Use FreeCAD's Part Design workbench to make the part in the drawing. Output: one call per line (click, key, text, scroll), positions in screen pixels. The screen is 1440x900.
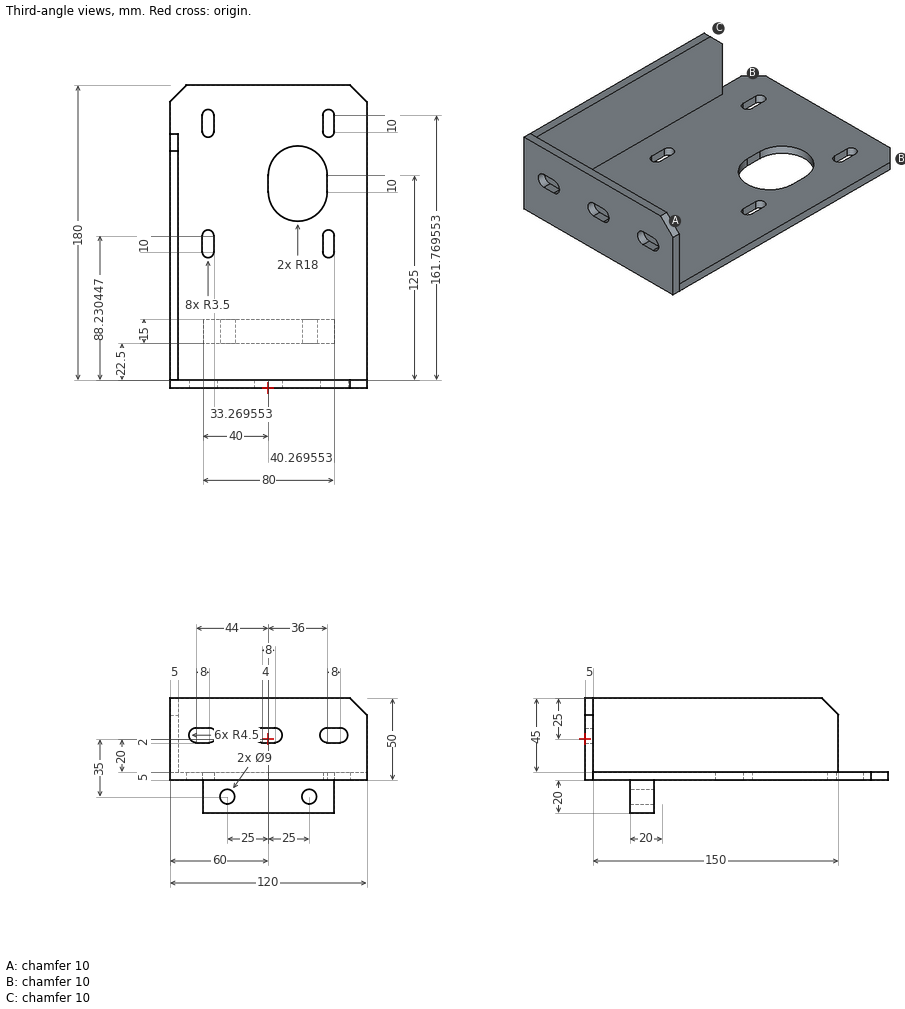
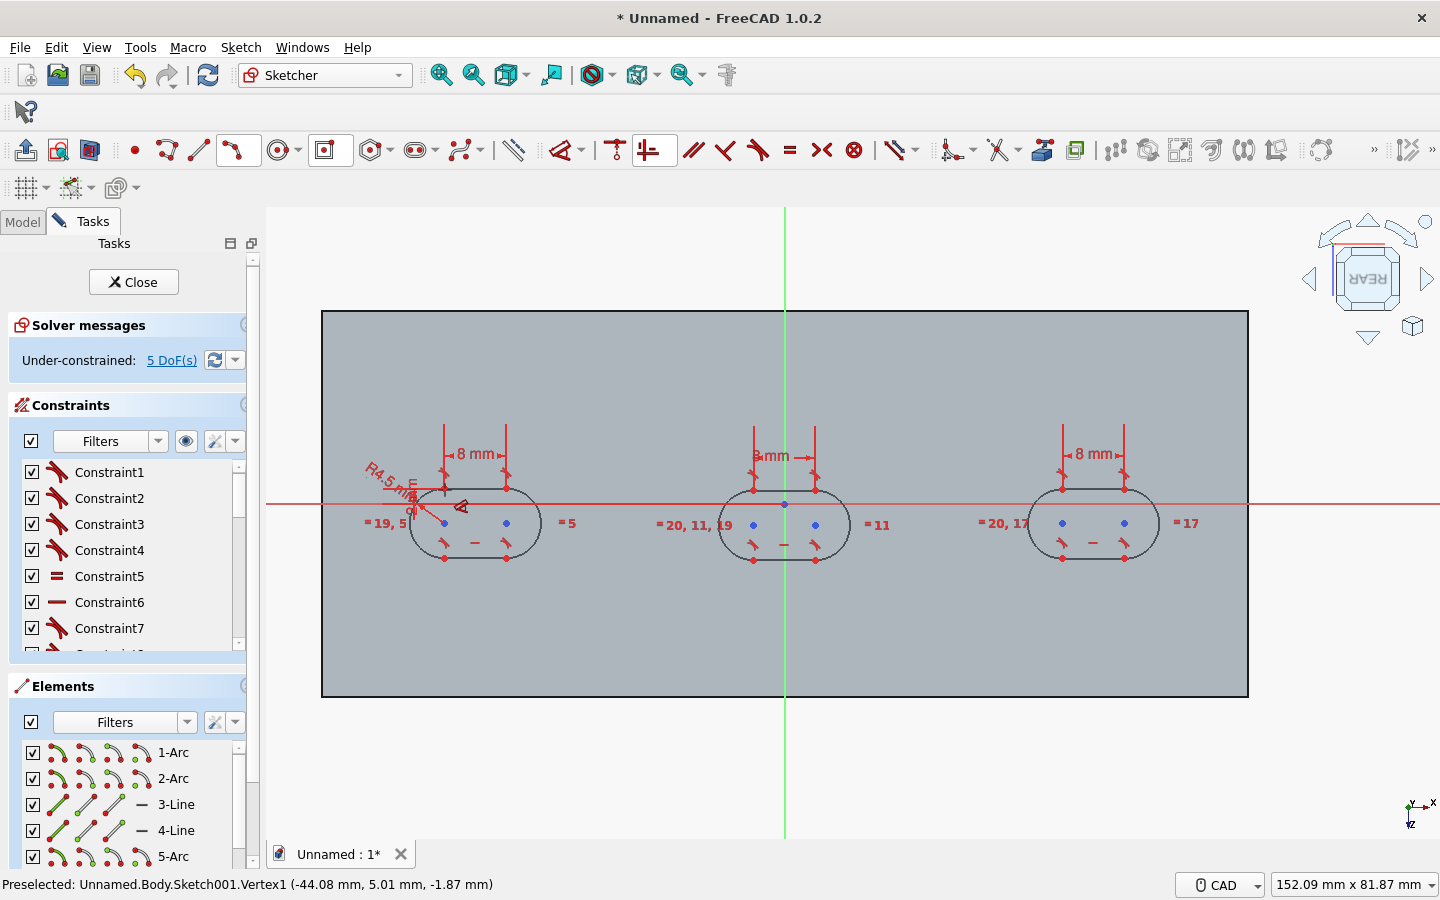
scroll(754, 491, up, 2)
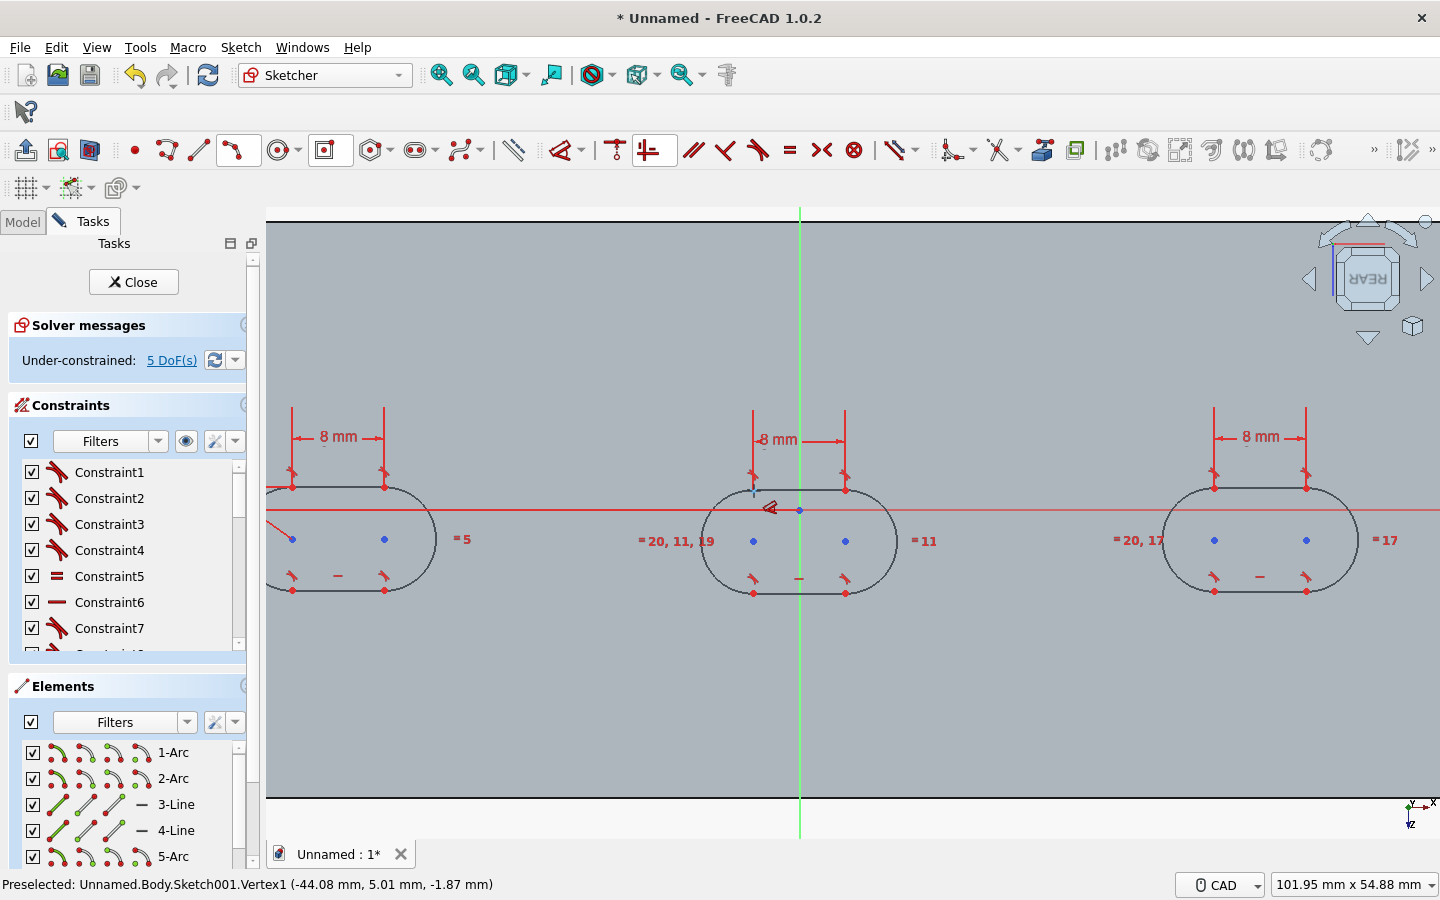
click(753, 490)
click(776, 544)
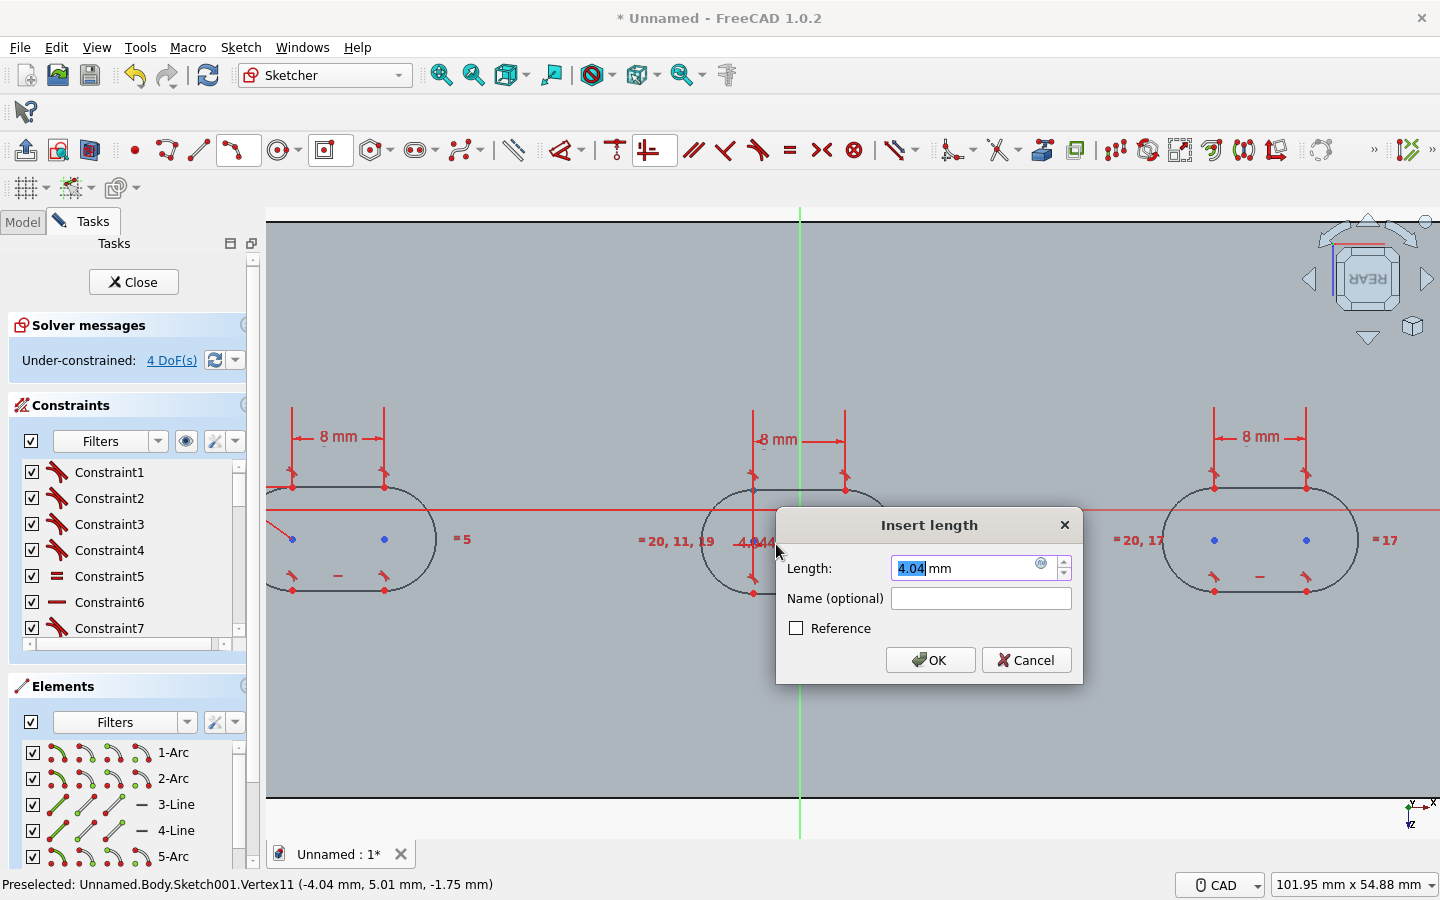
text(4)
key(Return)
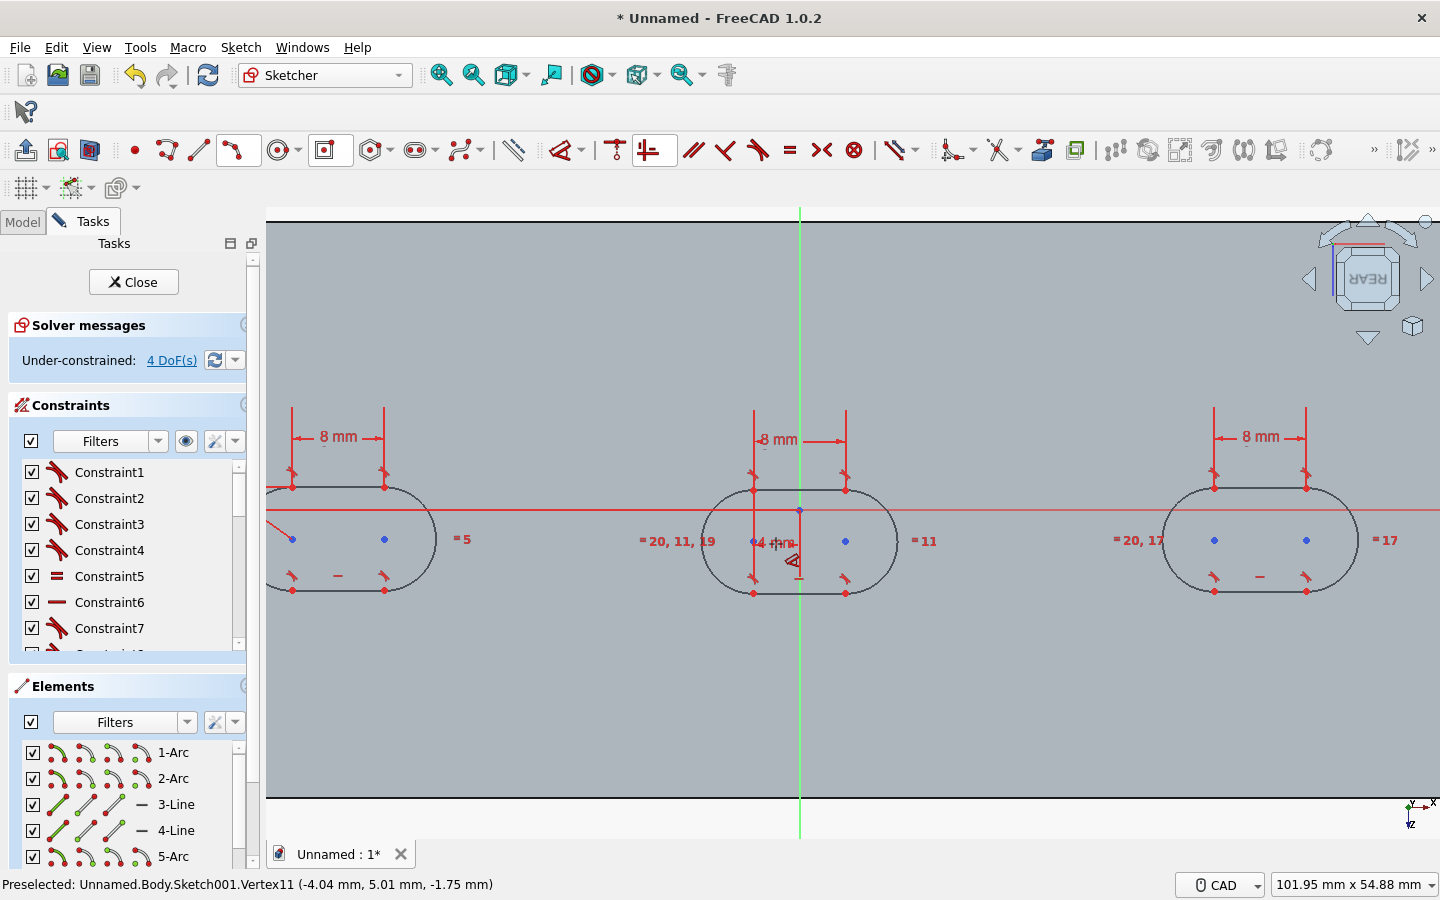
scroll(754, 490, up, 3)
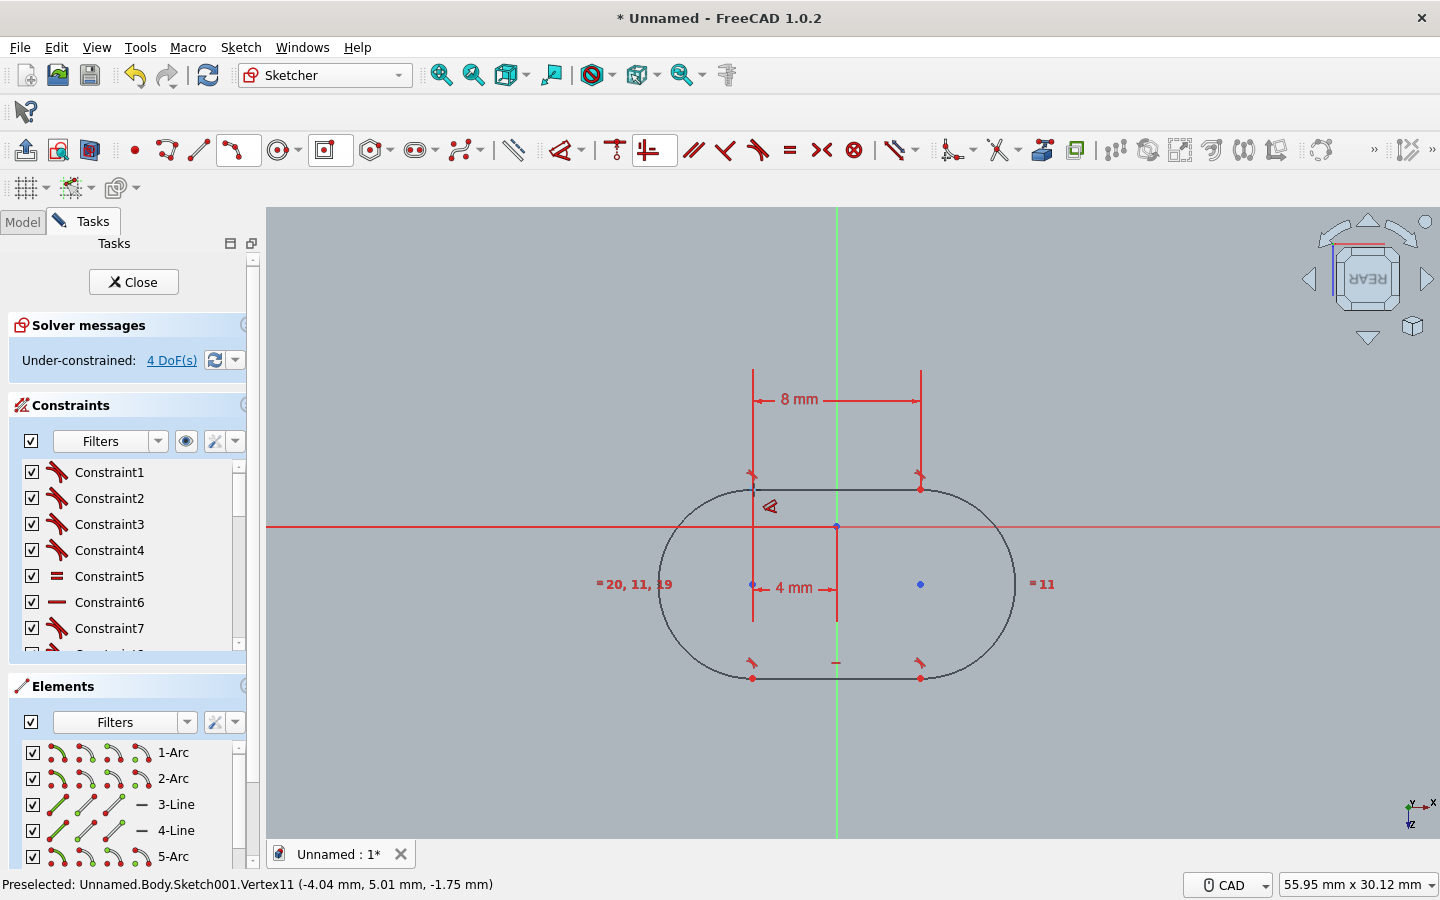
click(753, 490)
click(871, 508)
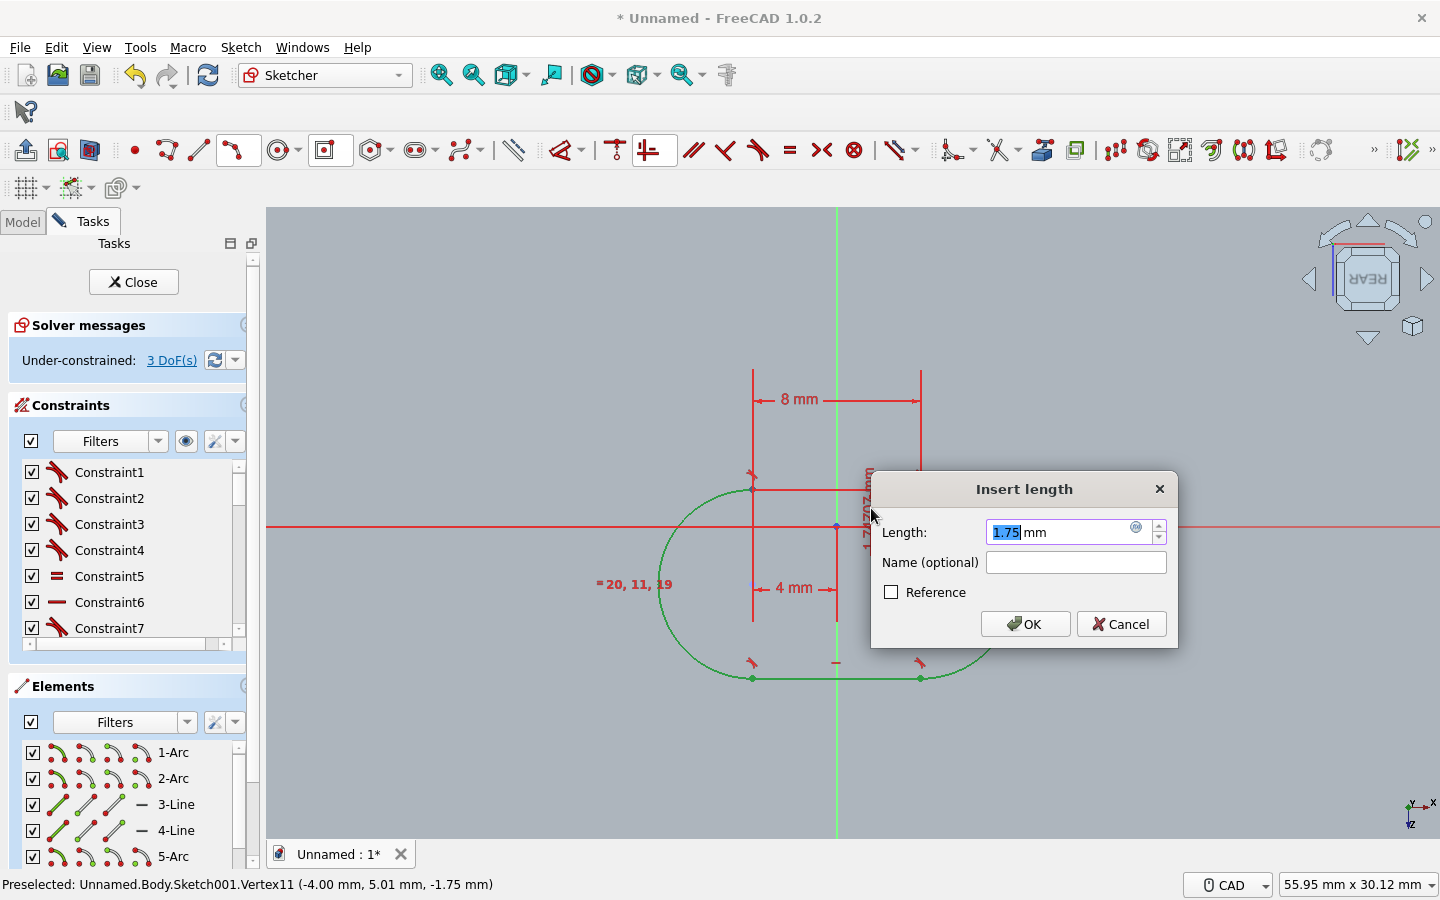
text(2)
key(Return)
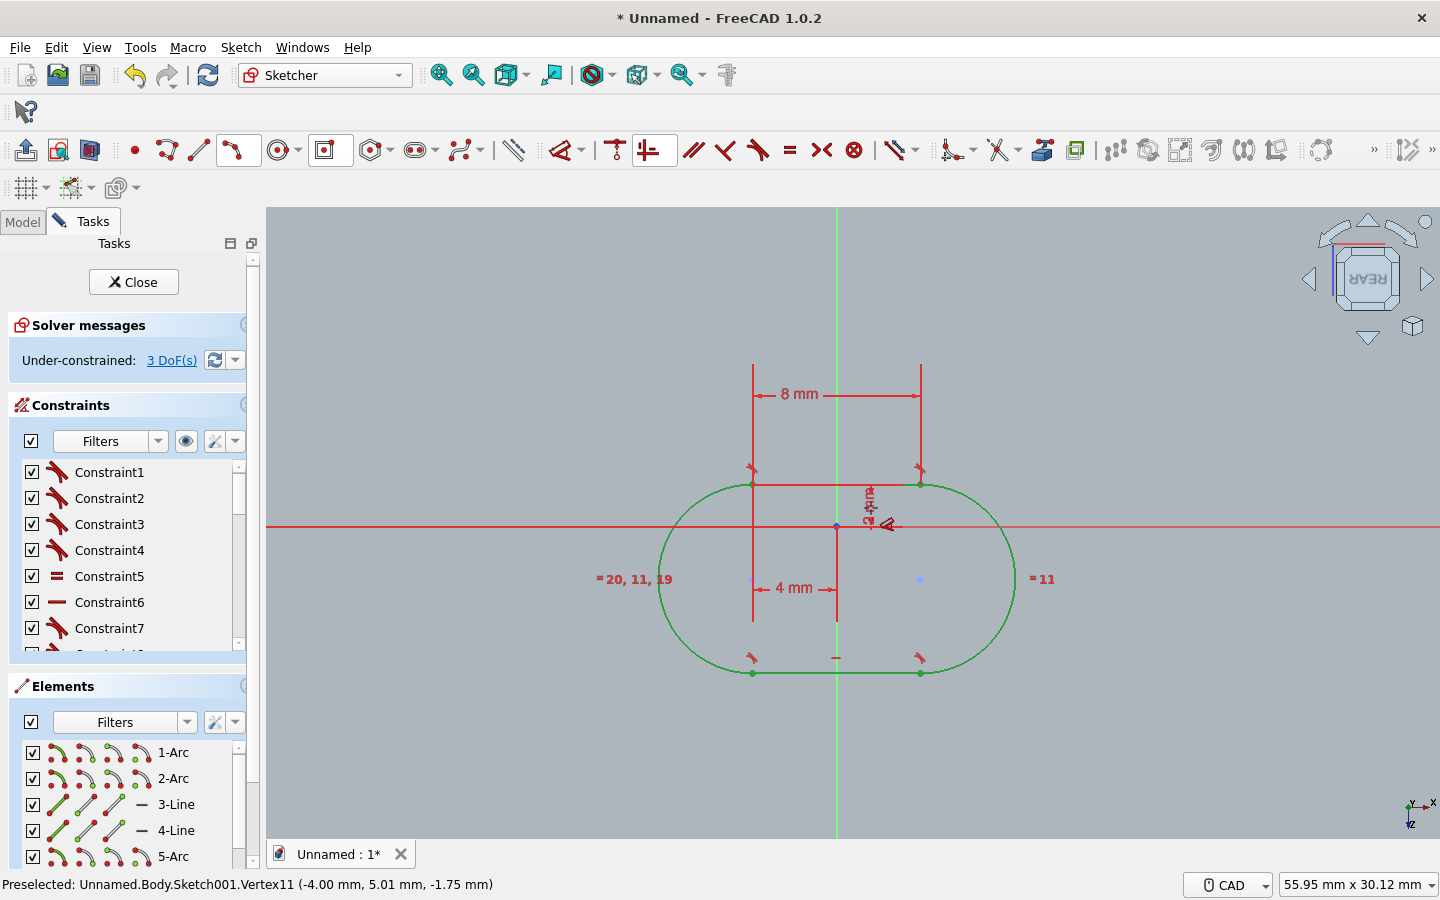
scroll(754, 490, down, 5)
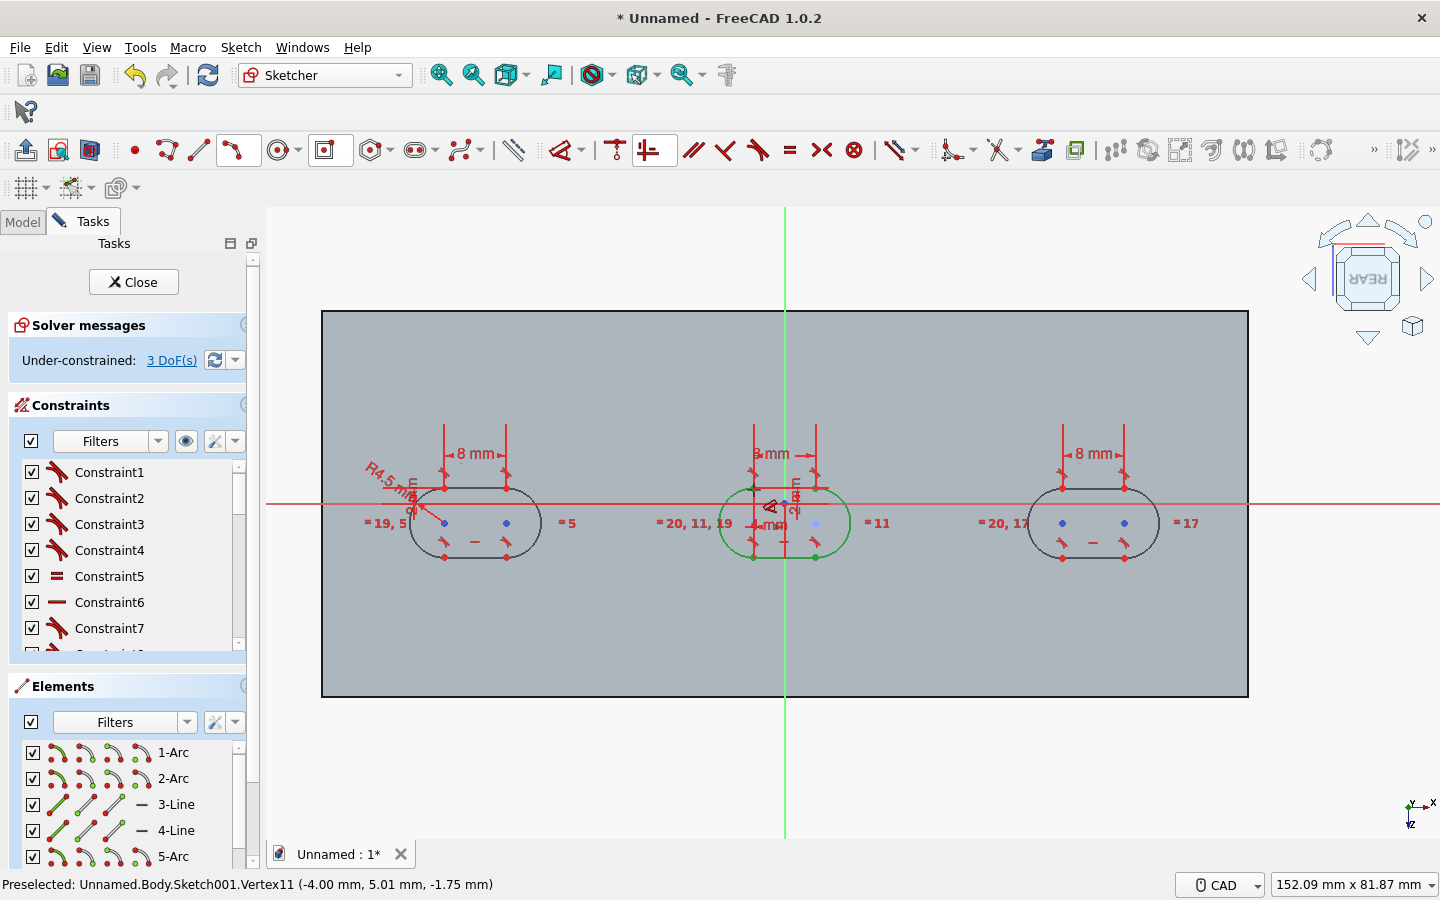
scroll(1063, 489, up, 5)